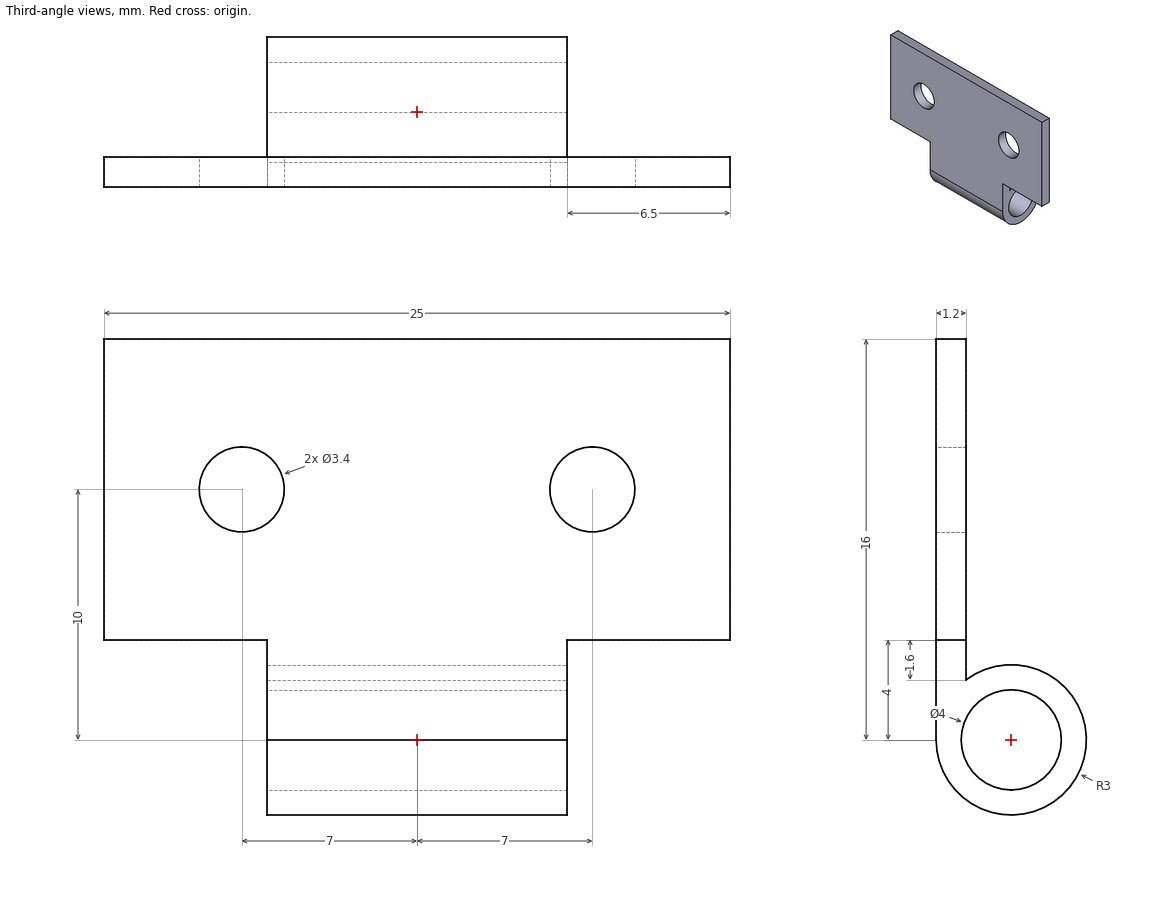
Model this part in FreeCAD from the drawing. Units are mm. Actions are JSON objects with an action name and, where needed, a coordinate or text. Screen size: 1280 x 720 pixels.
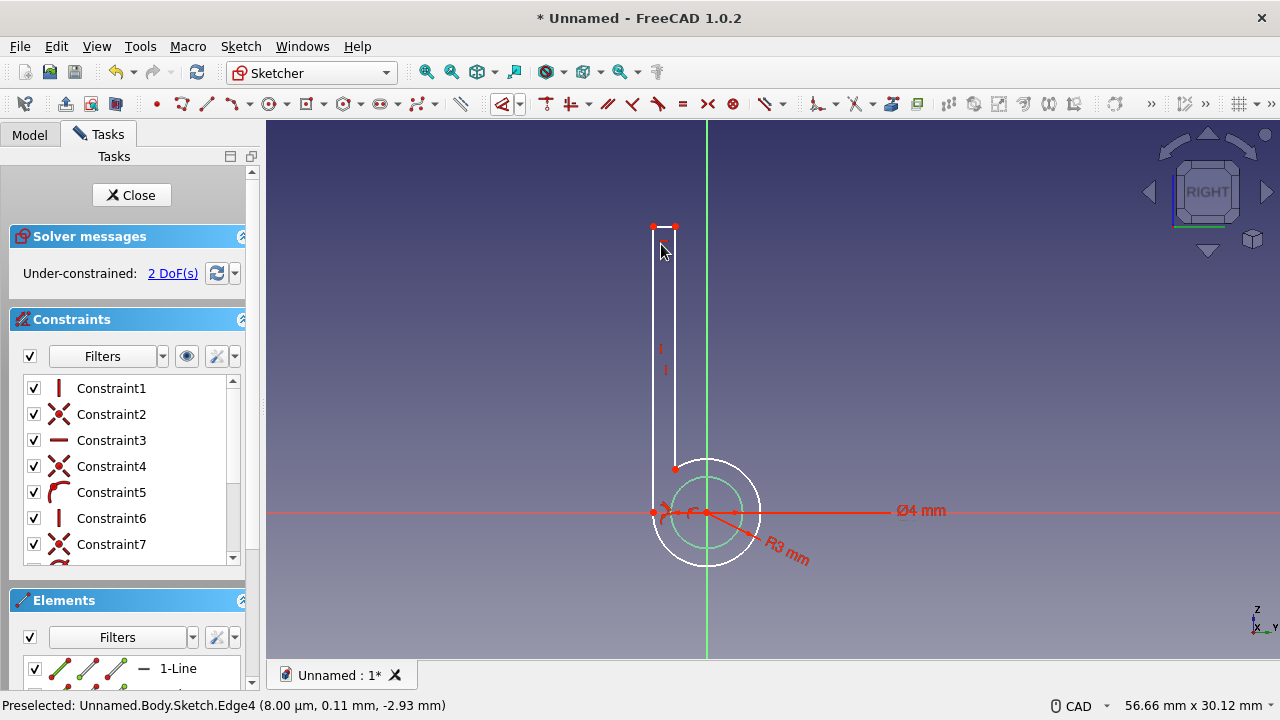
{"action": "left_click", "coordinate": [653, 313]}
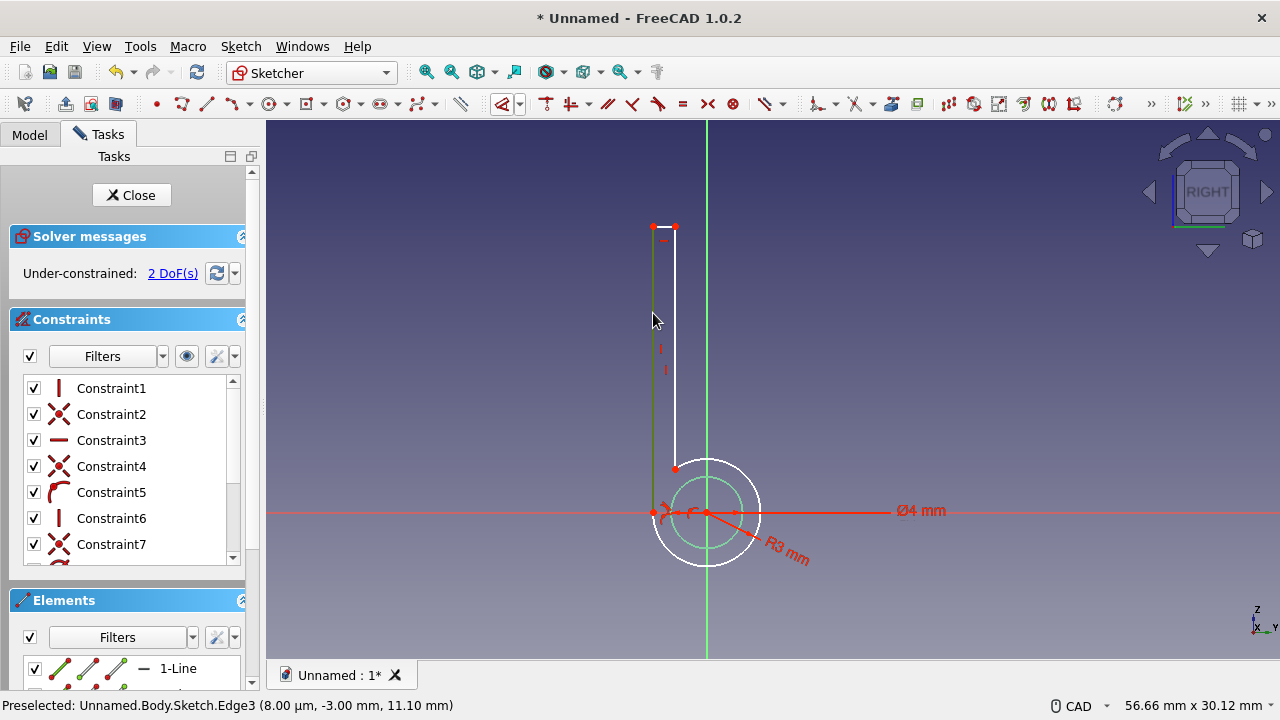
{"action": "key", "text": "i"}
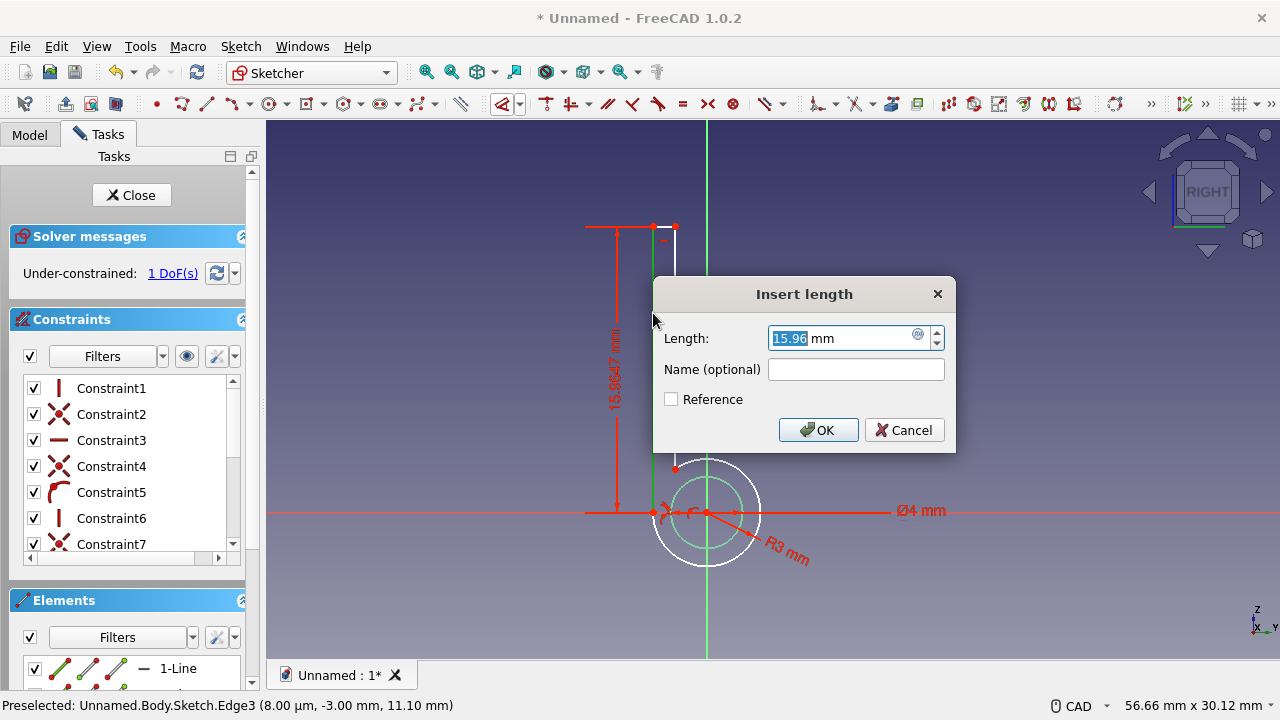
{"action": "type", "text": "16"}
{"action": "key", "text": "Return"}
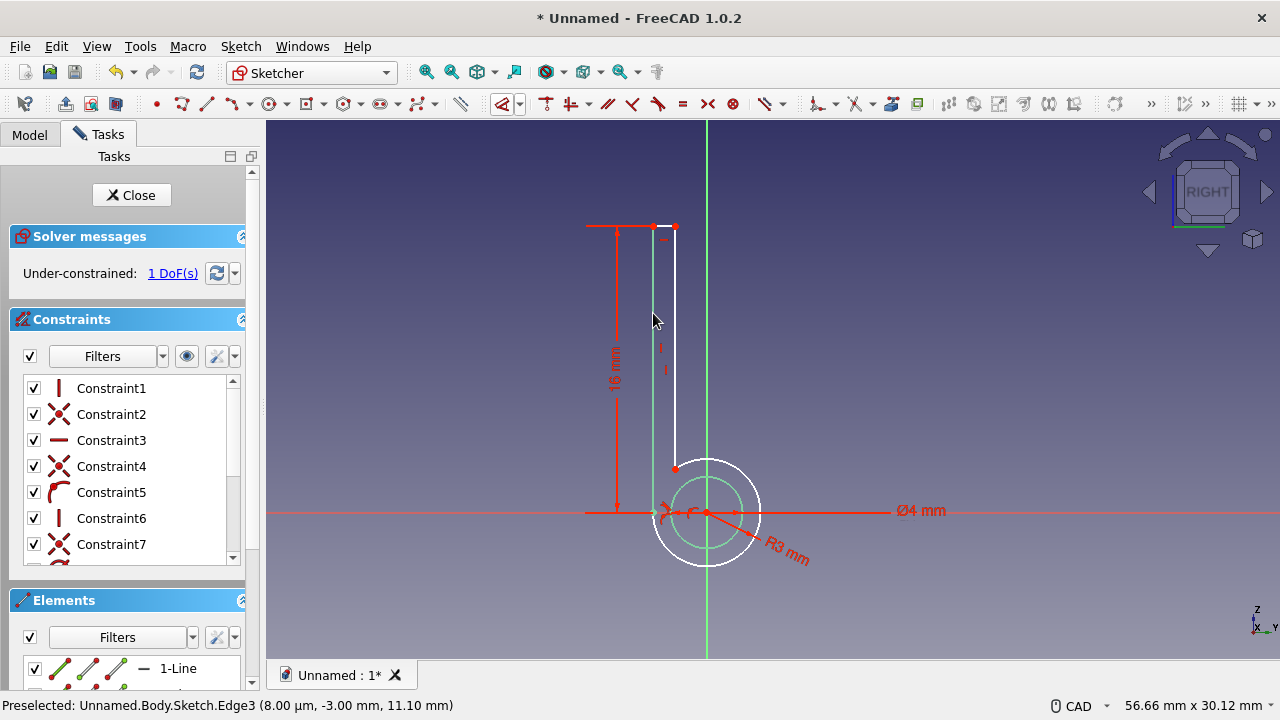
{"action": "scroll", "coordinate": [664, 226], "scroll_direction": "up", "scroll_amount": 4}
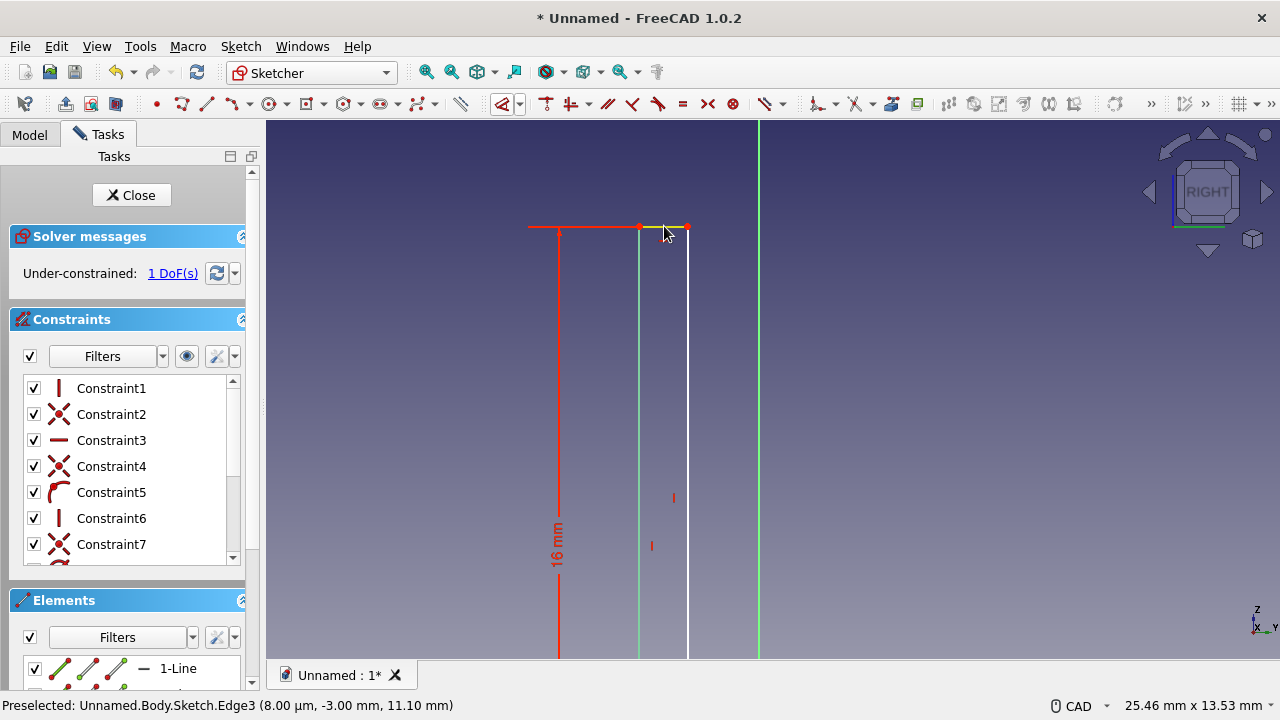
{"action": "left_click", "coordinate": [664, 227]}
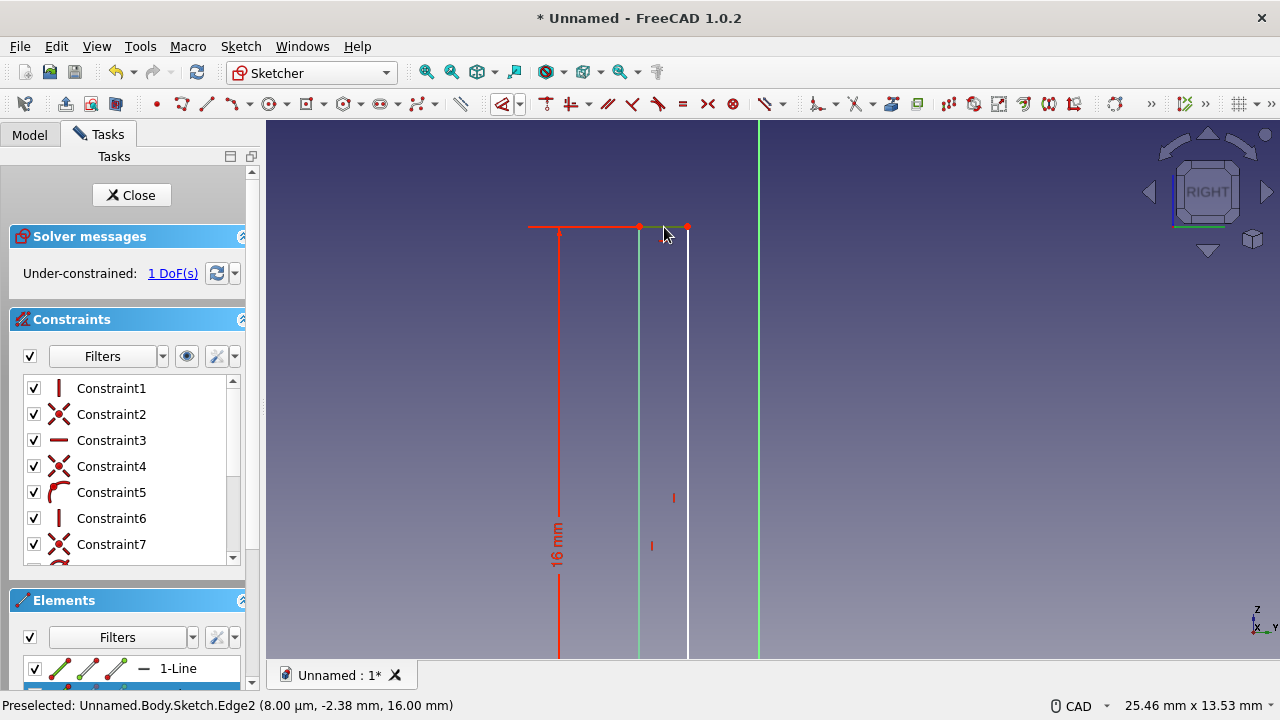
{"action": "left_click", "coordinate": [520, 104]}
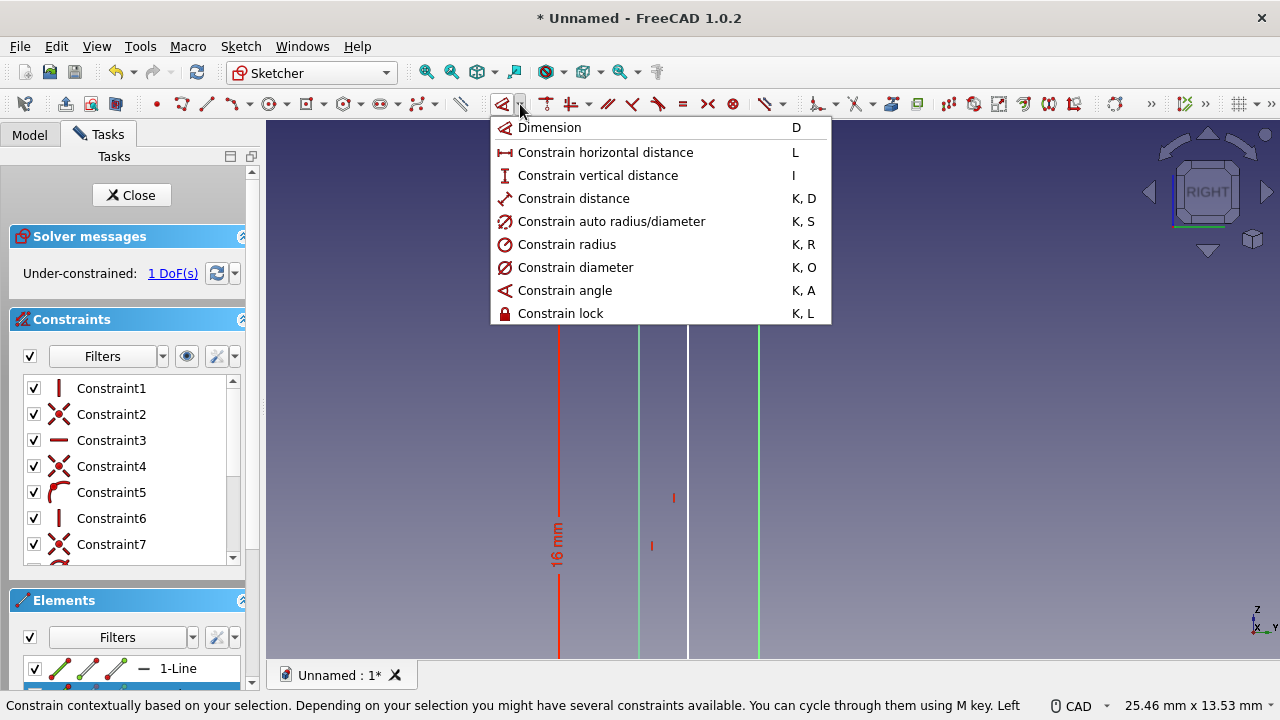
{"action": "left_click", "coordinate": [661, 152]}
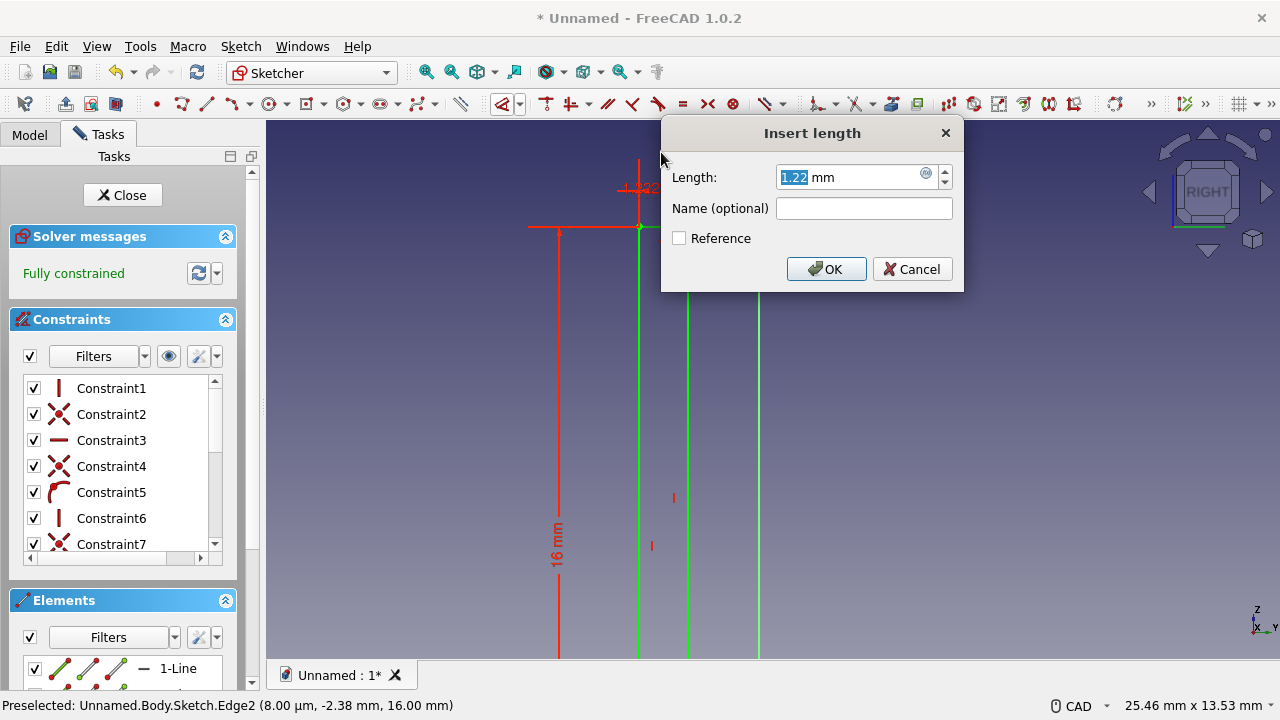
{"action": "type", "text": "1.2"}
{"action": "key", "text": "Return"}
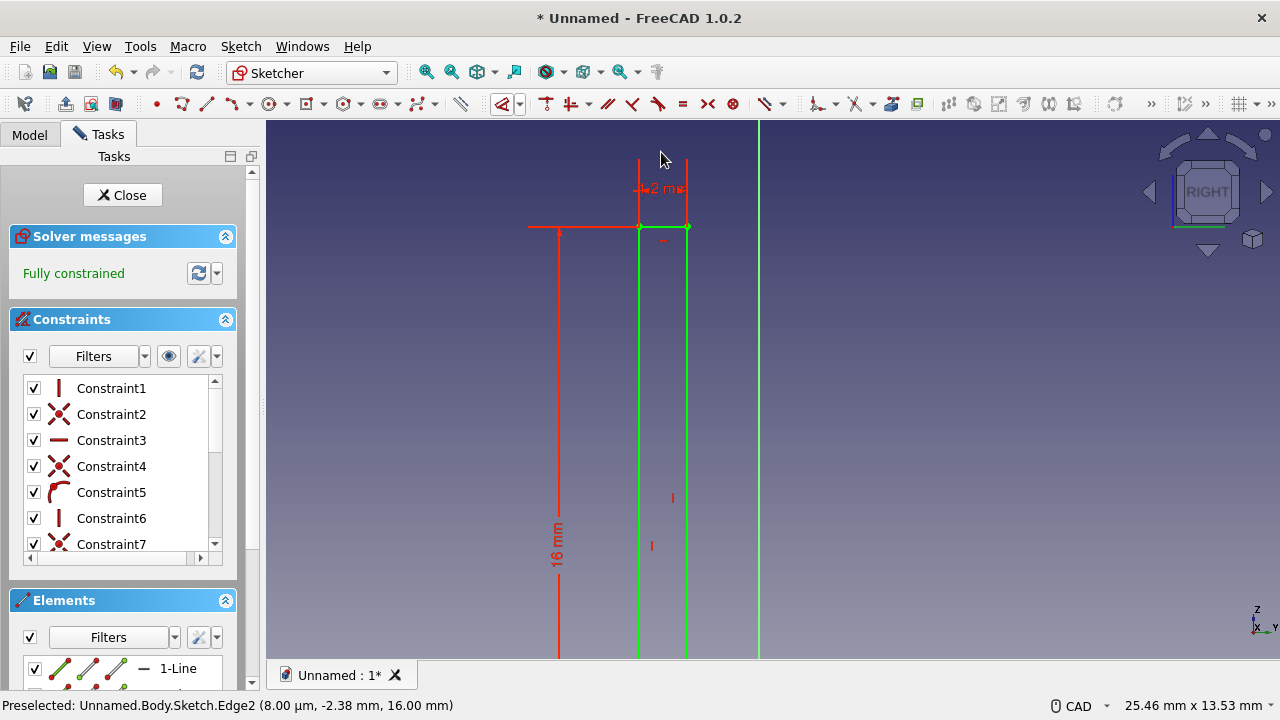
{"action": "left_click", "coordinate": [123, 195]}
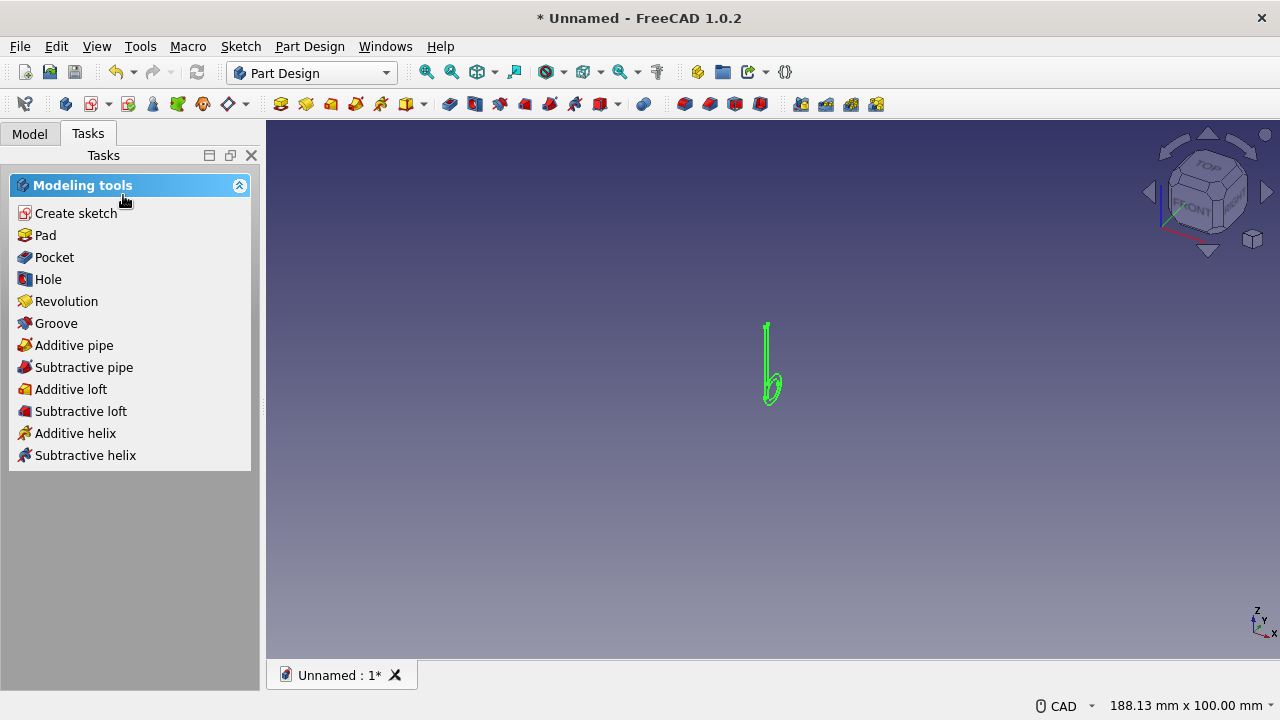
{"action": "left_click", "coordinate": [281, 104]}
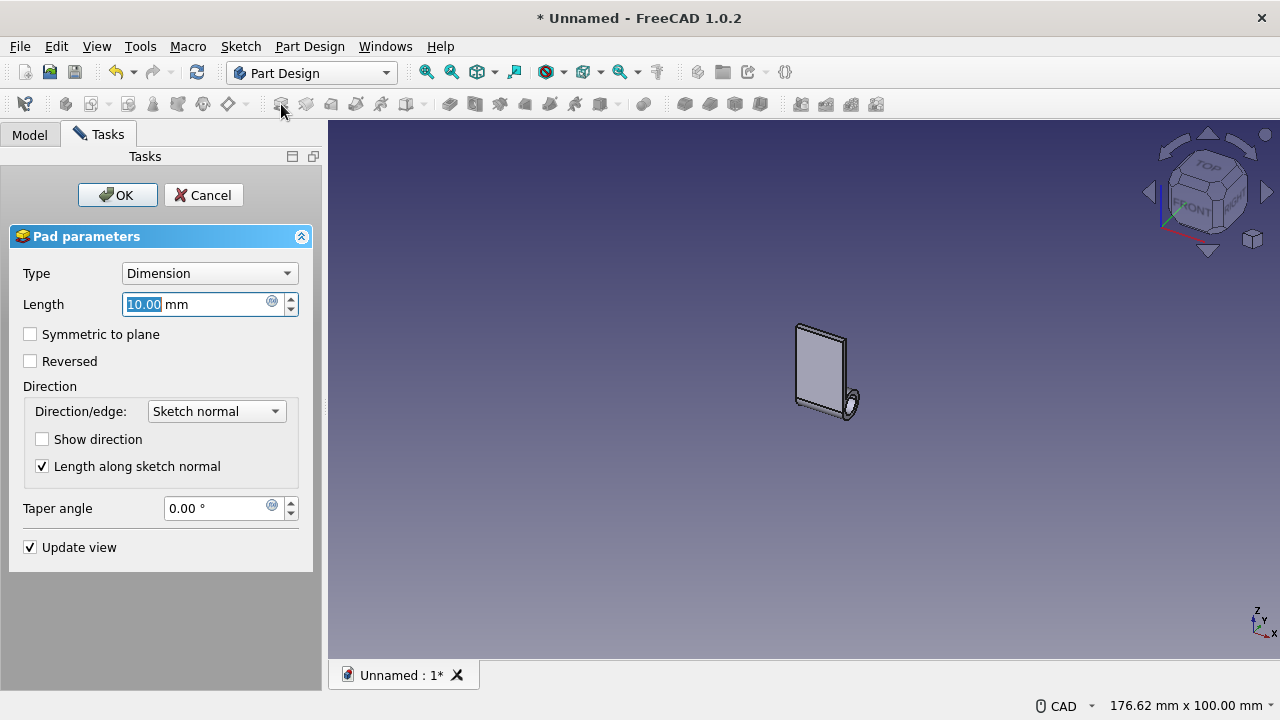
{"action": "type", "text": "25"}
{"action": "key", "text": "Tab"}